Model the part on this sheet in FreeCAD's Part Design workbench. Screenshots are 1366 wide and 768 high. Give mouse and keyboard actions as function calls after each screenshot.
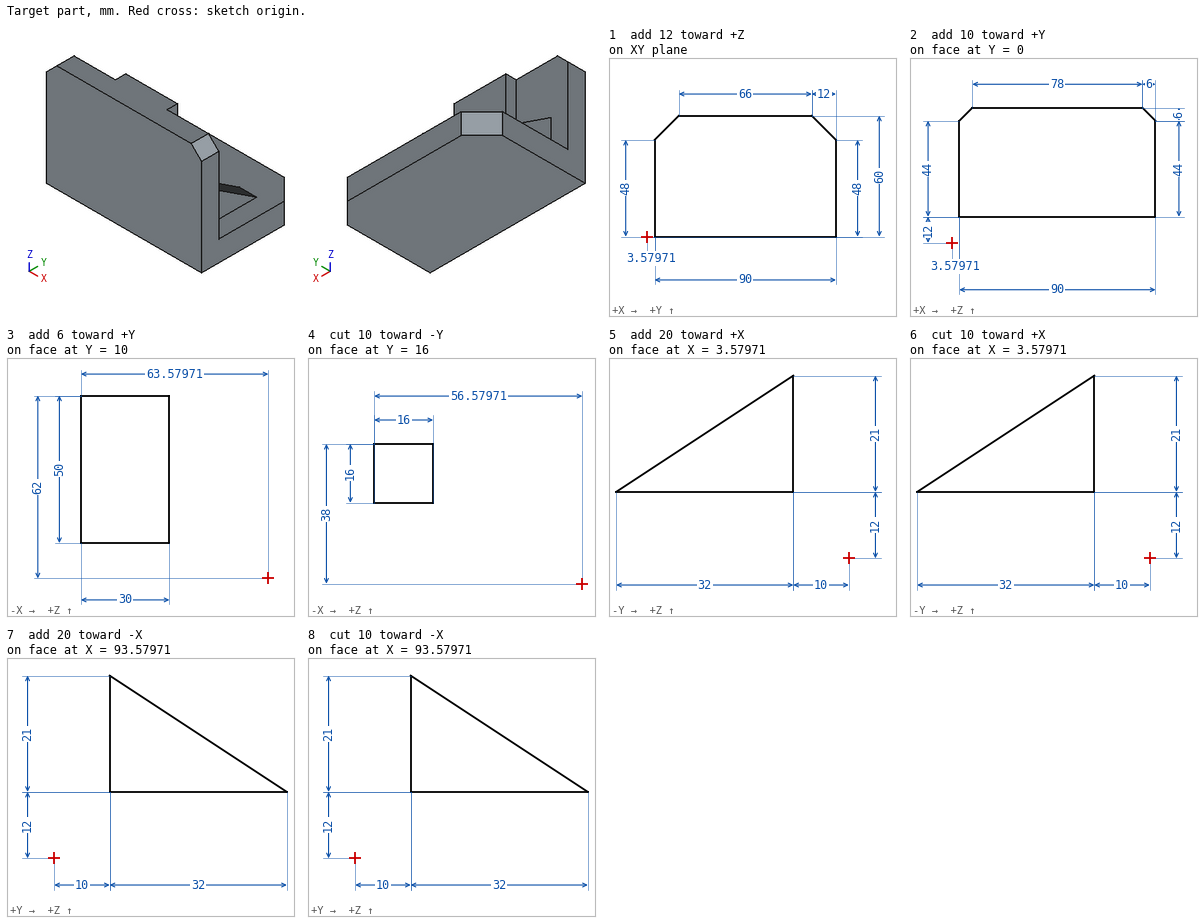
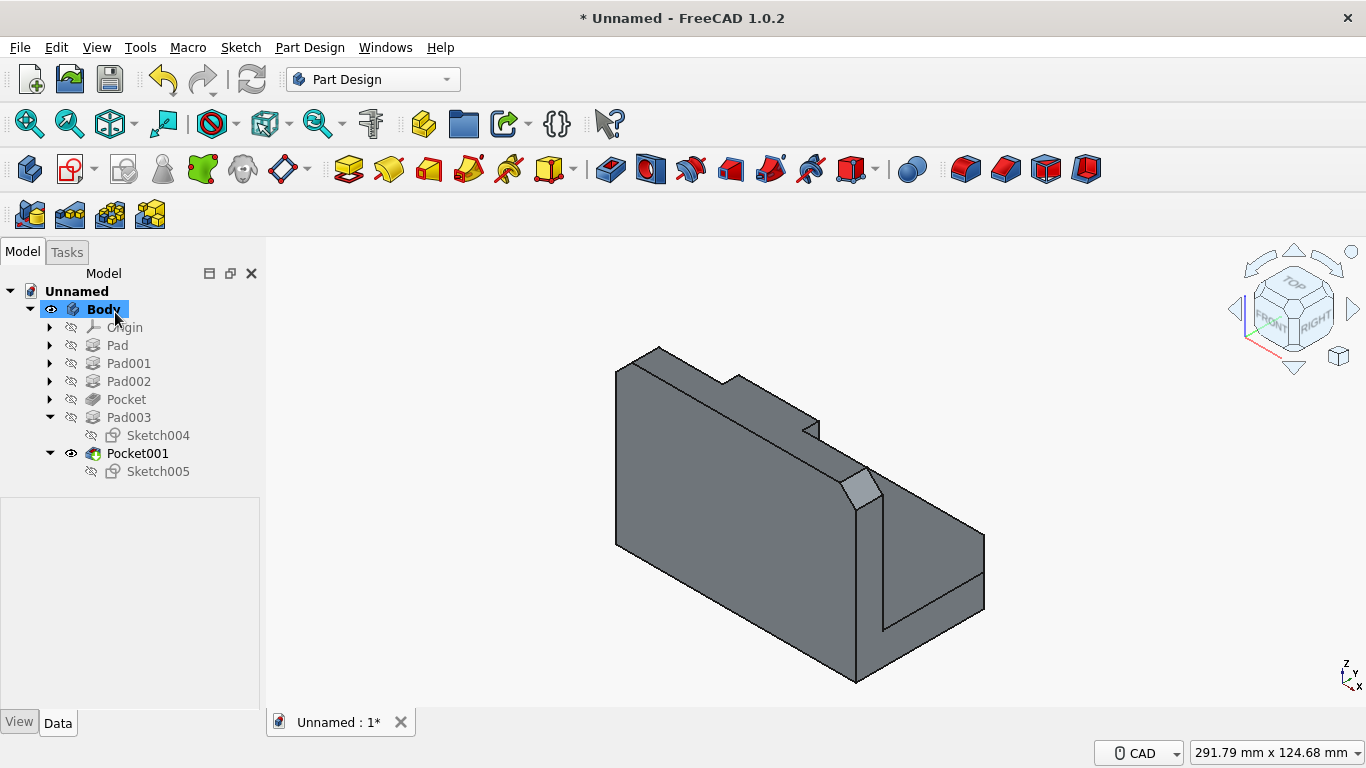
click(957, 611)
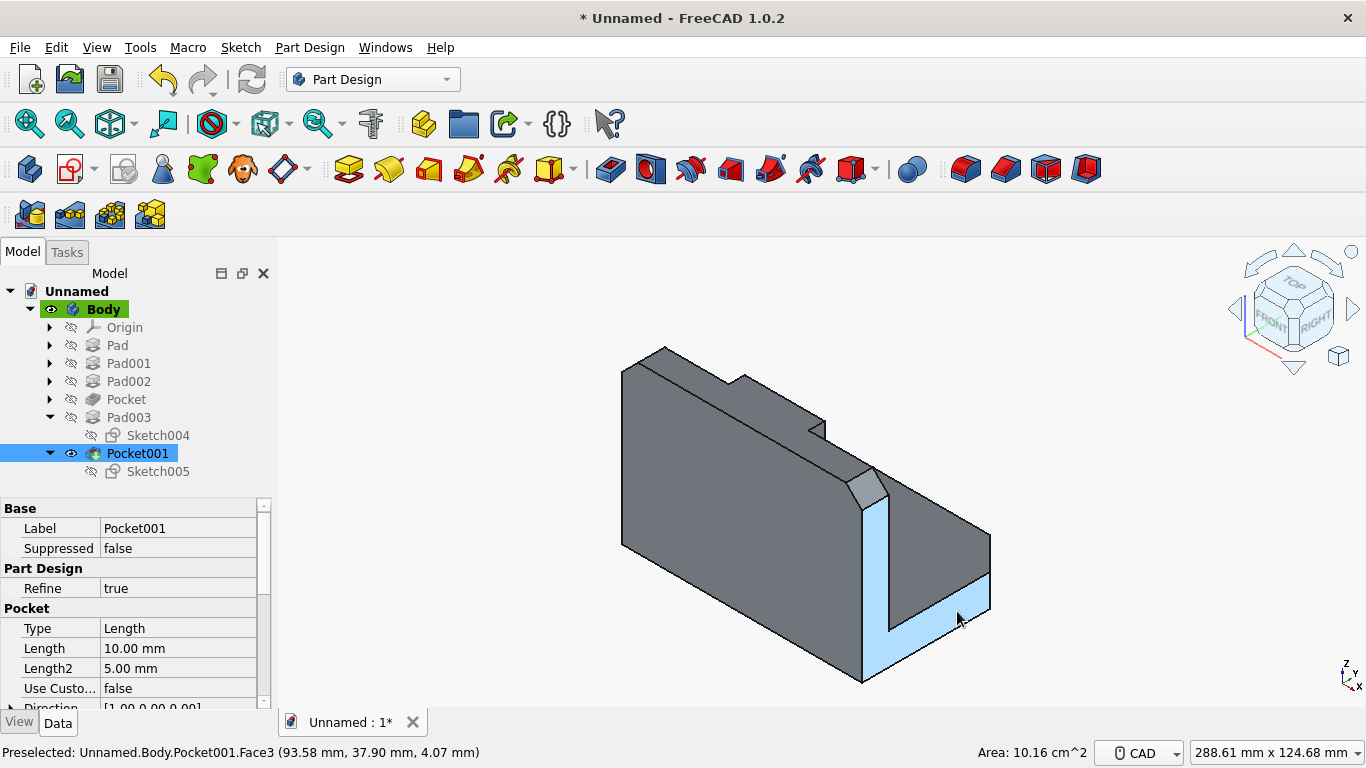
click(70, 170)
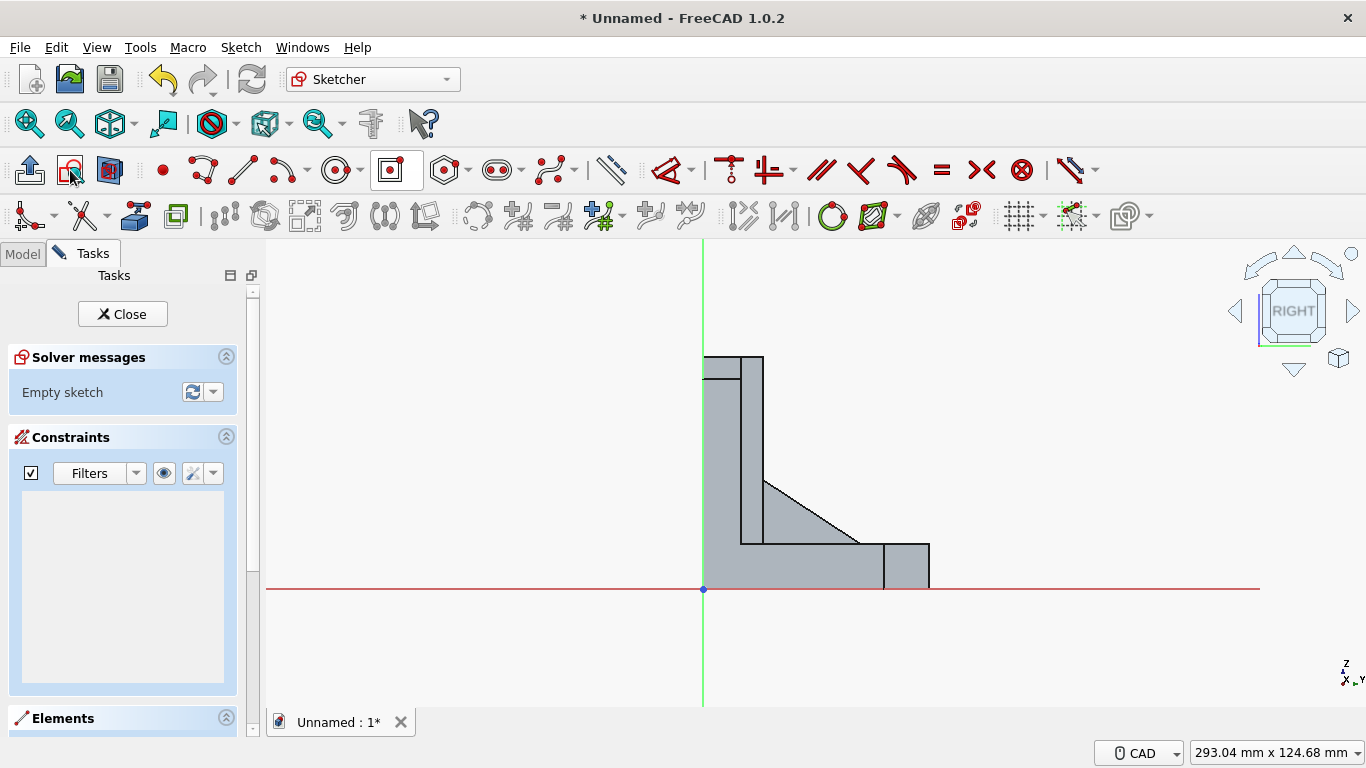
scroll(811, 572, up, 4)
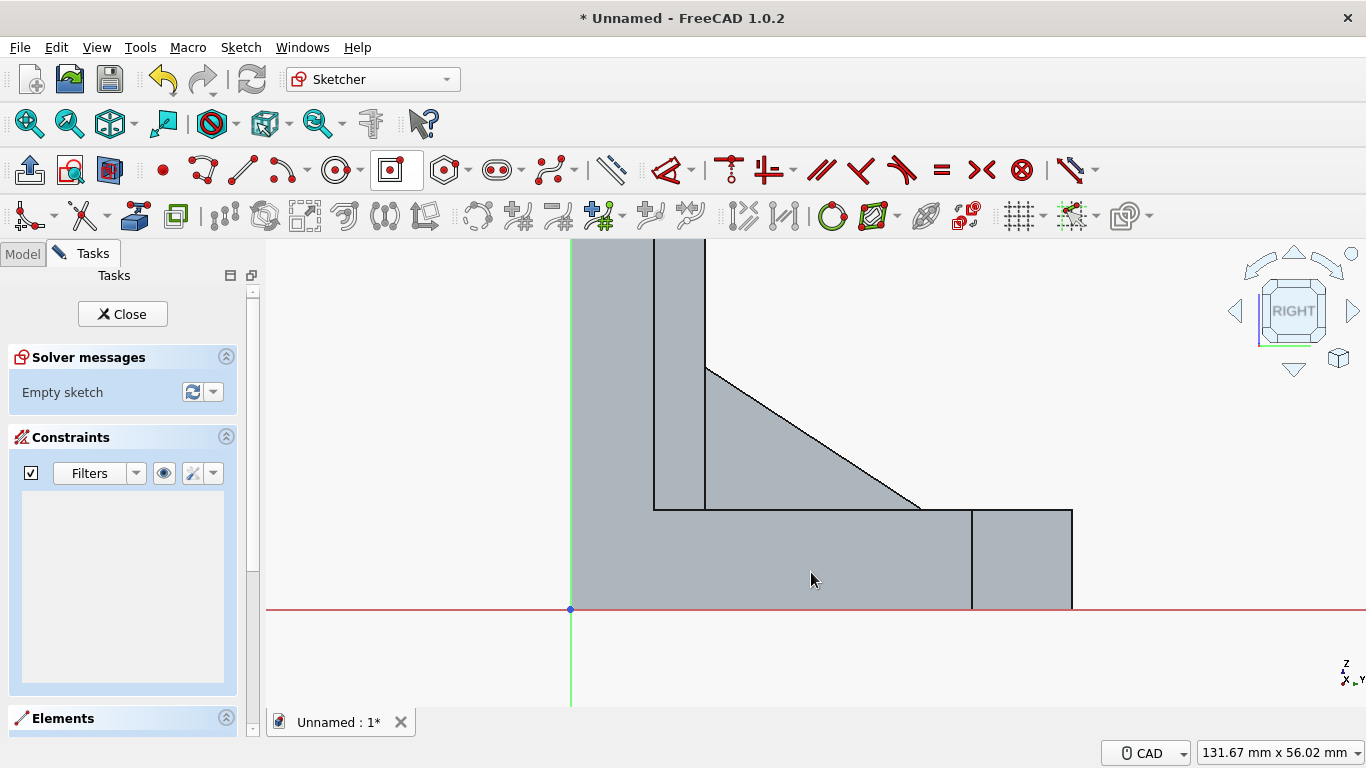
key(g)
key(m)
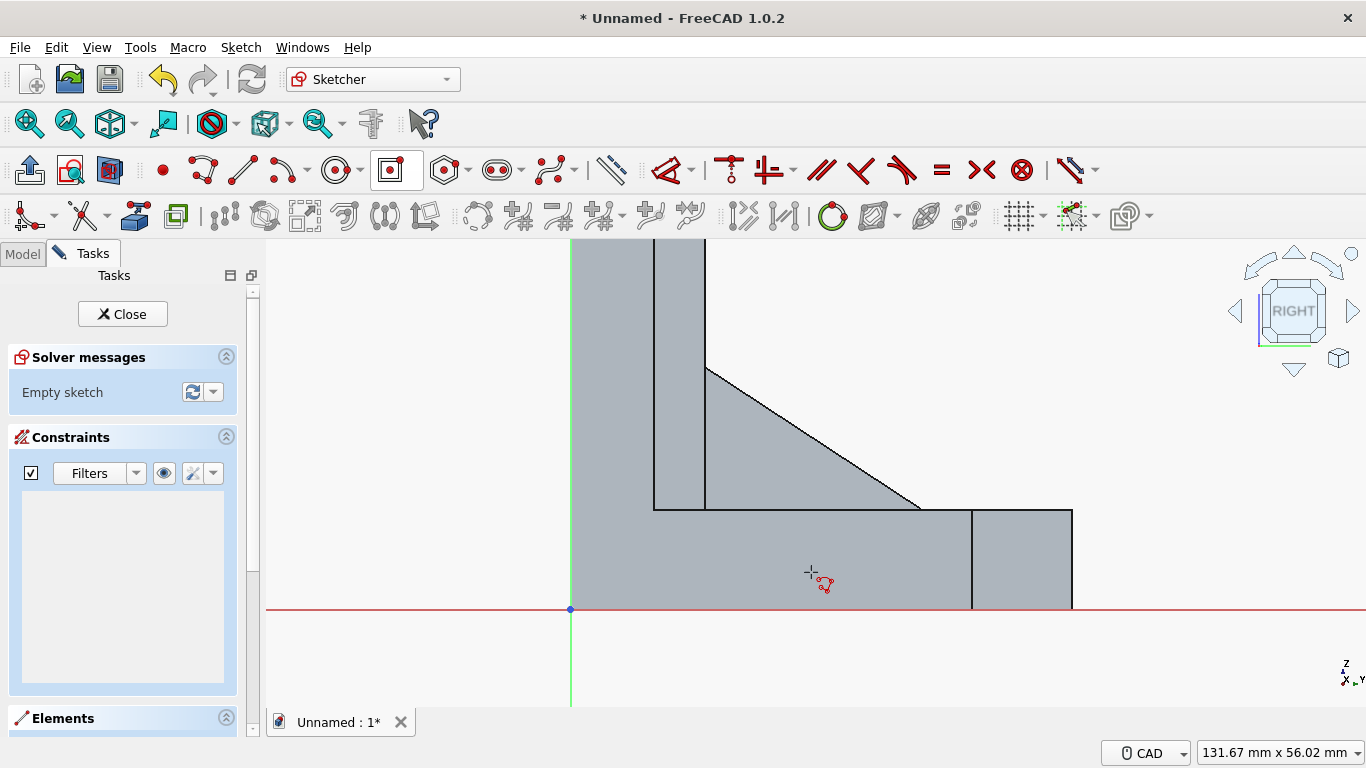
click(654, 510)
click(922, 510)
click(654, 334)
click(654, 511)
key(Escape)
key(Escape)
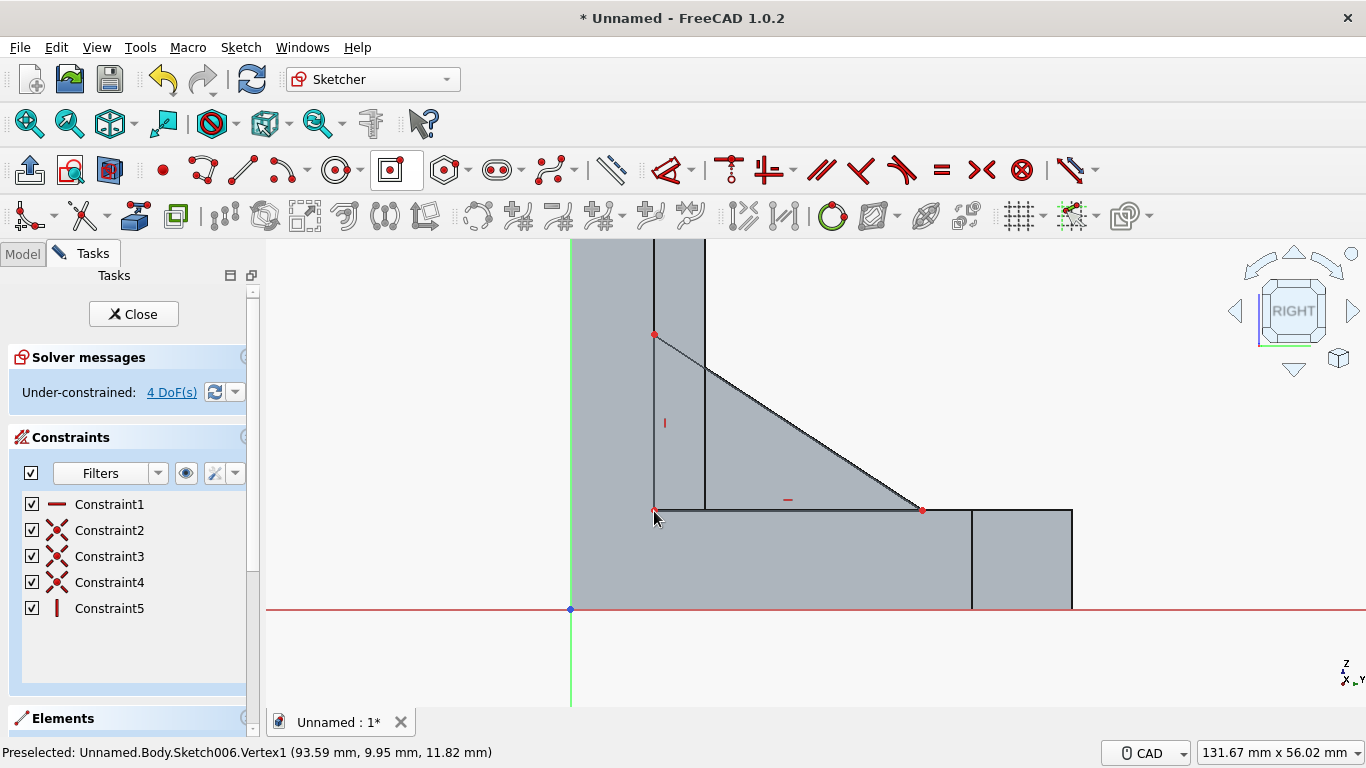
click(666, 170)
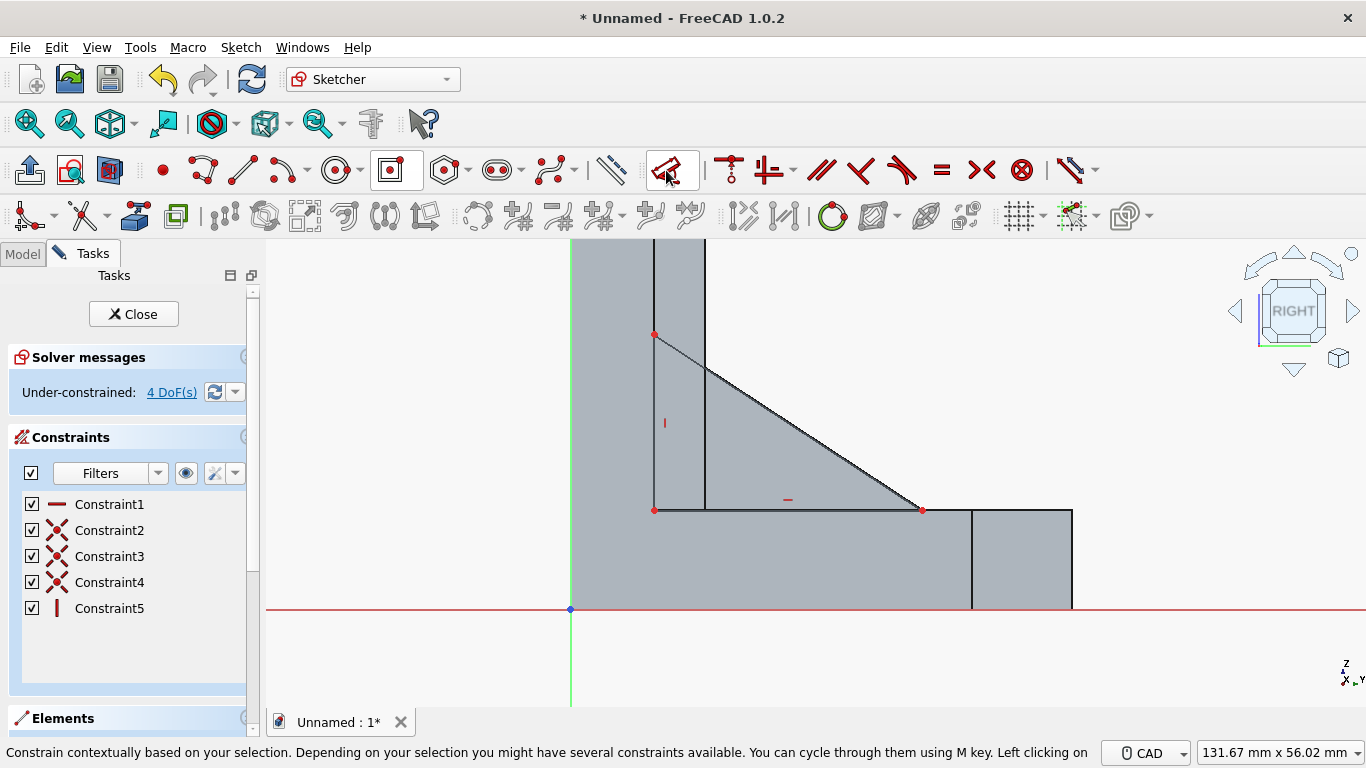
click(734, 511)
click(788, 545)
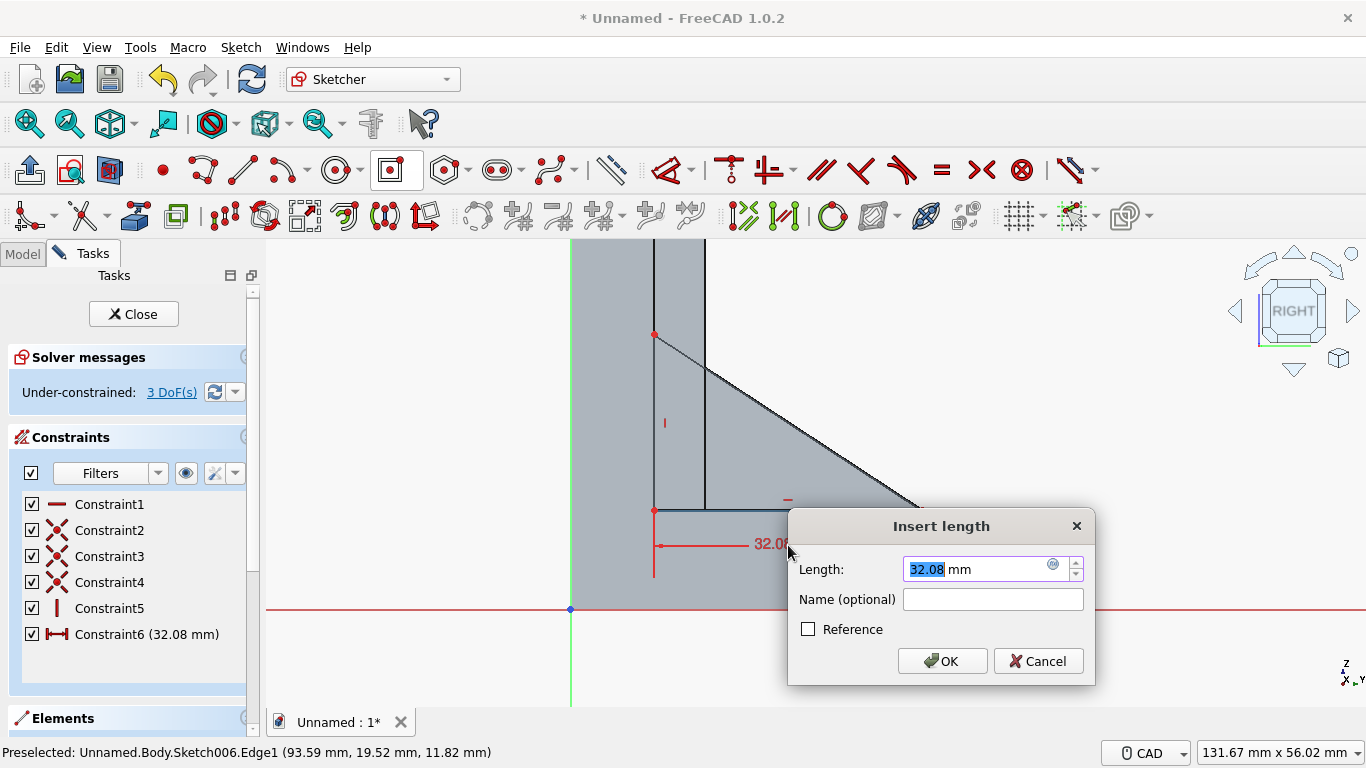
text(32)
key(Return)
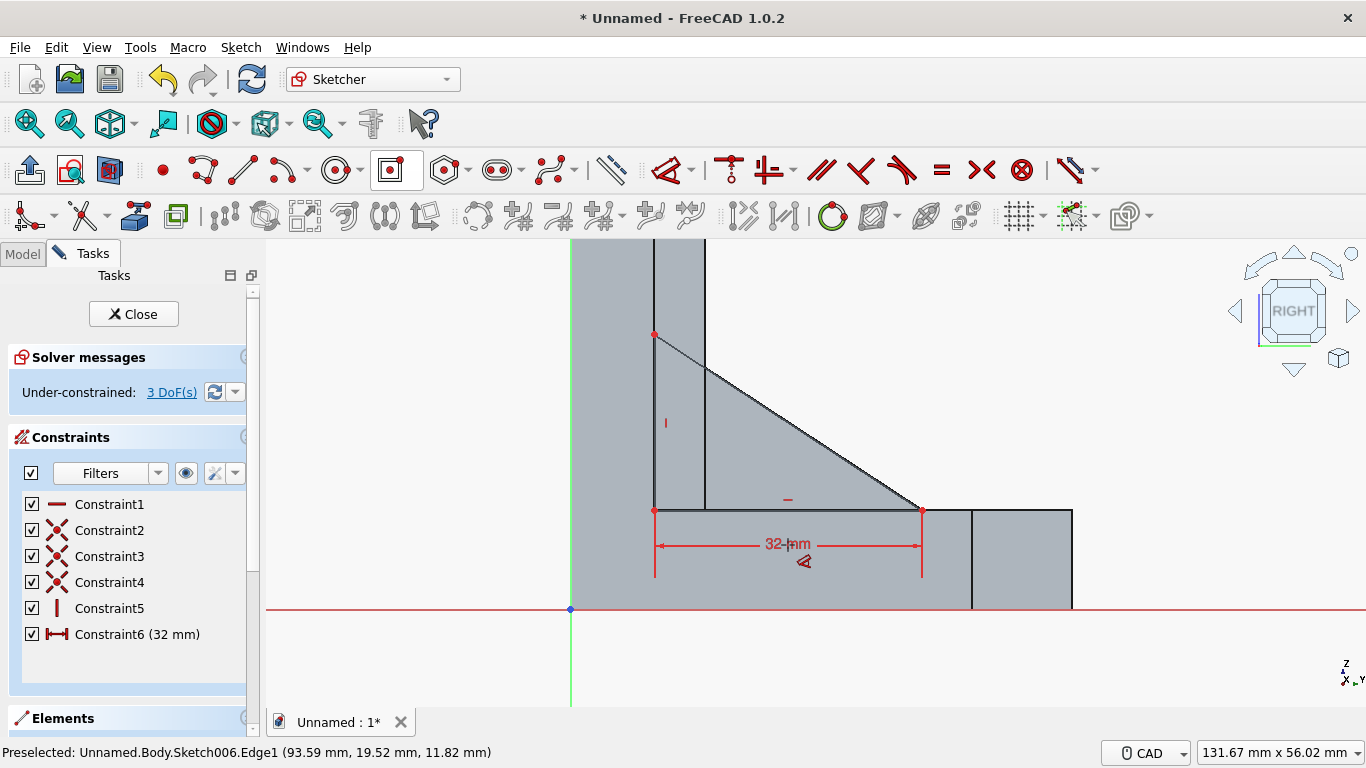
click(655, 388)
click(621, 423)